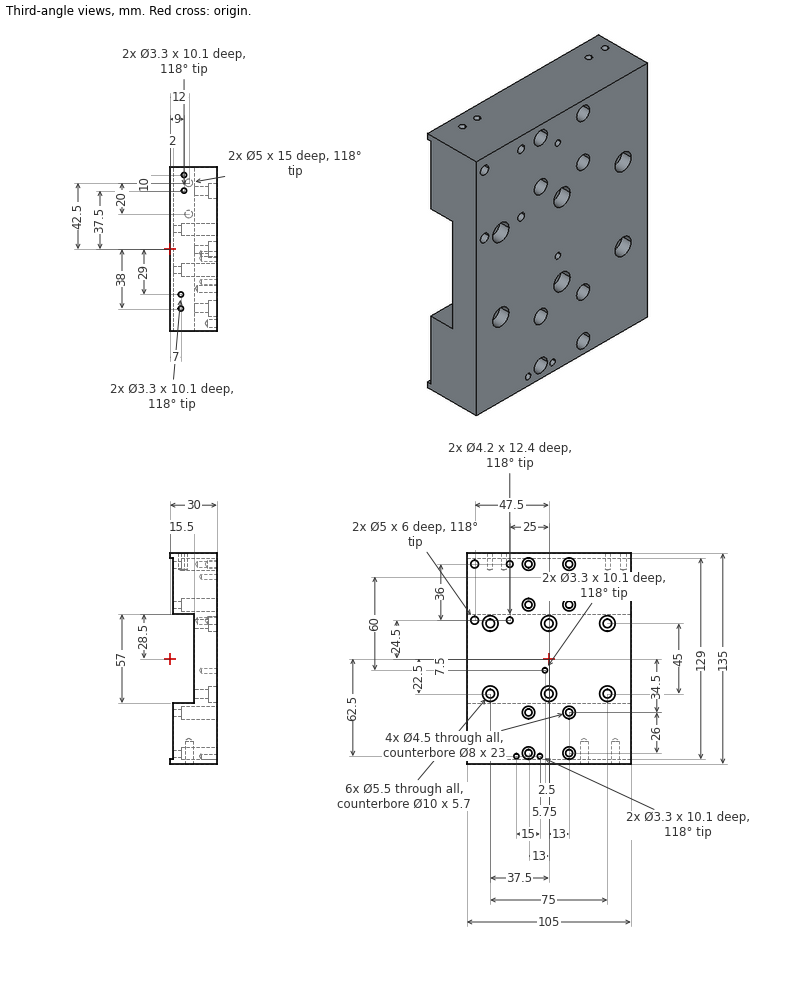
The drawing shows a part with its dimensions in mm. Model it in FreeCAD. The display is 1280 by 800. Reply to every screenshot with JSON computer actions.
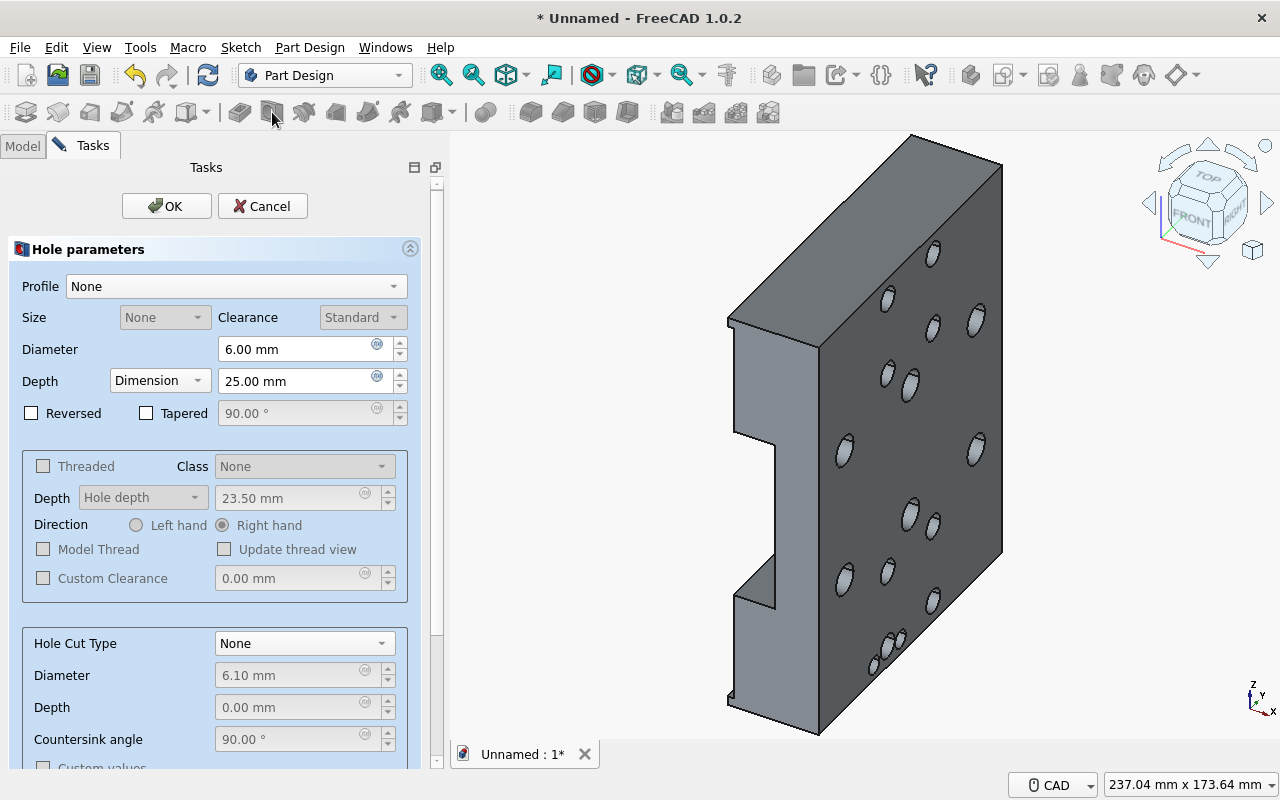
{"action": "triple_click", "coordinate": [305, 349]}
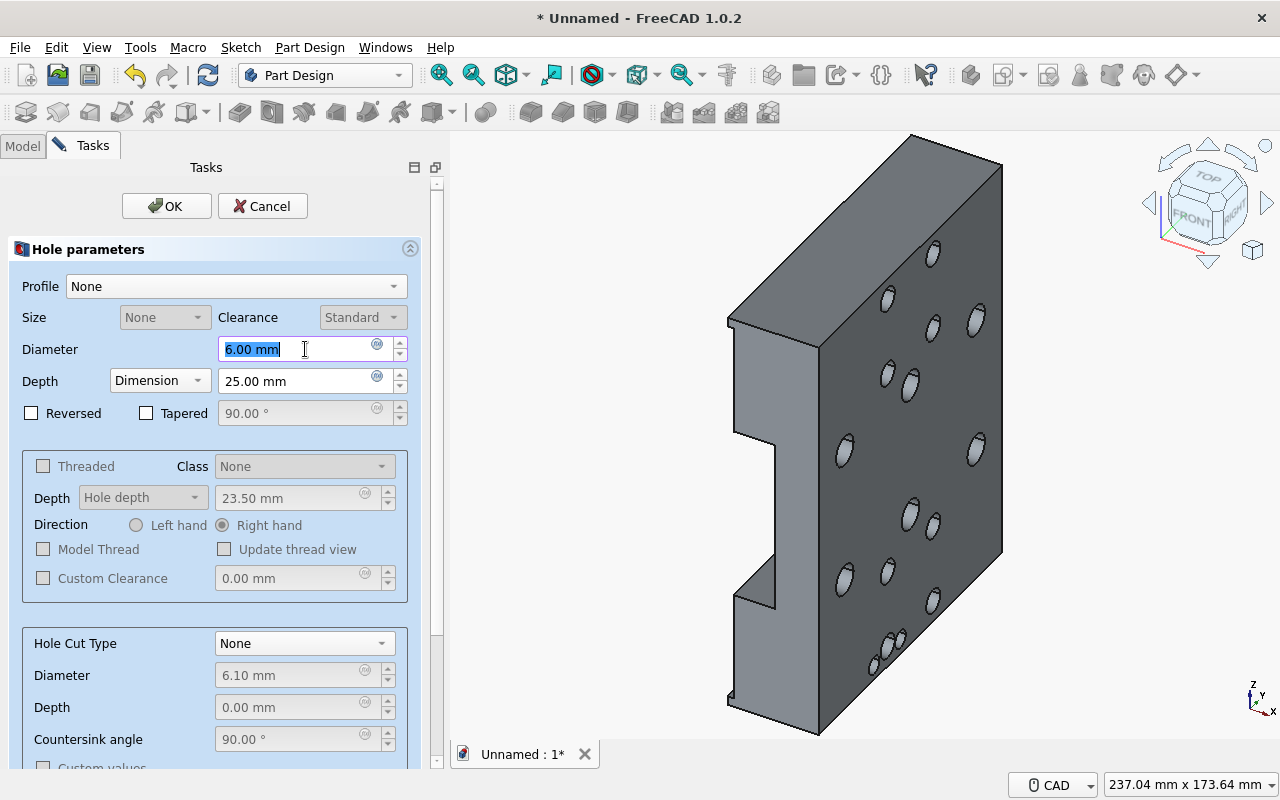
{"action": "type", "text": "3.3"}
{"action": "key", "text": "Tab"}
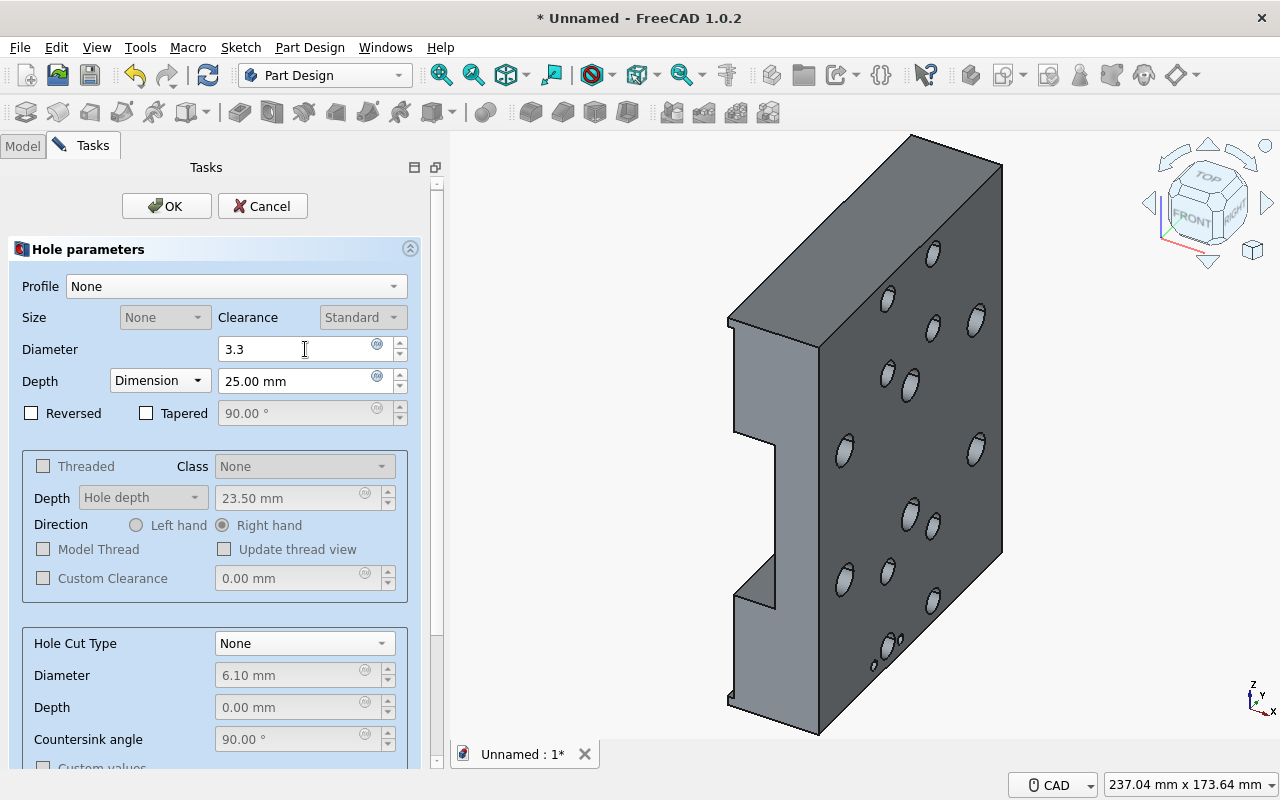
{"action": "triple_click", "coordinate": [305, 381]}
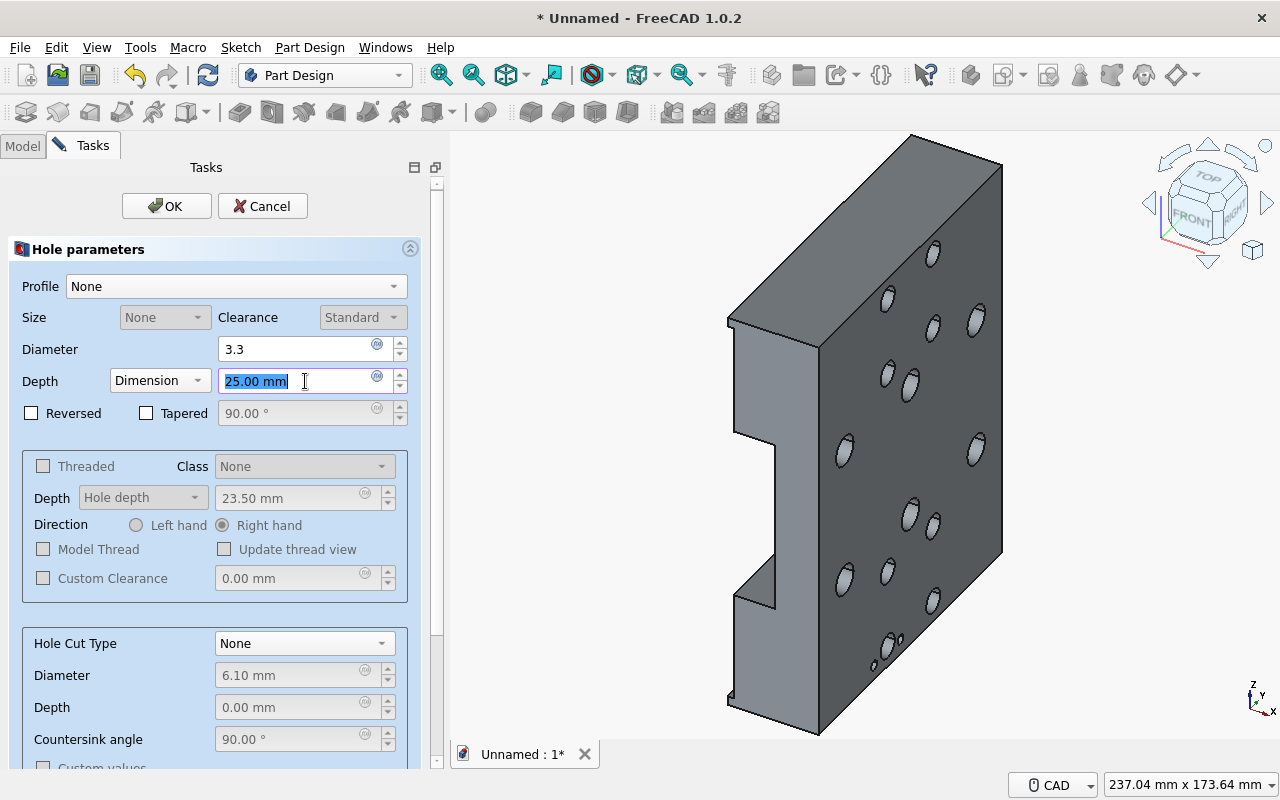
{"action": "type", "text": "10.1"}
{"action": "key", "text": "Tab"}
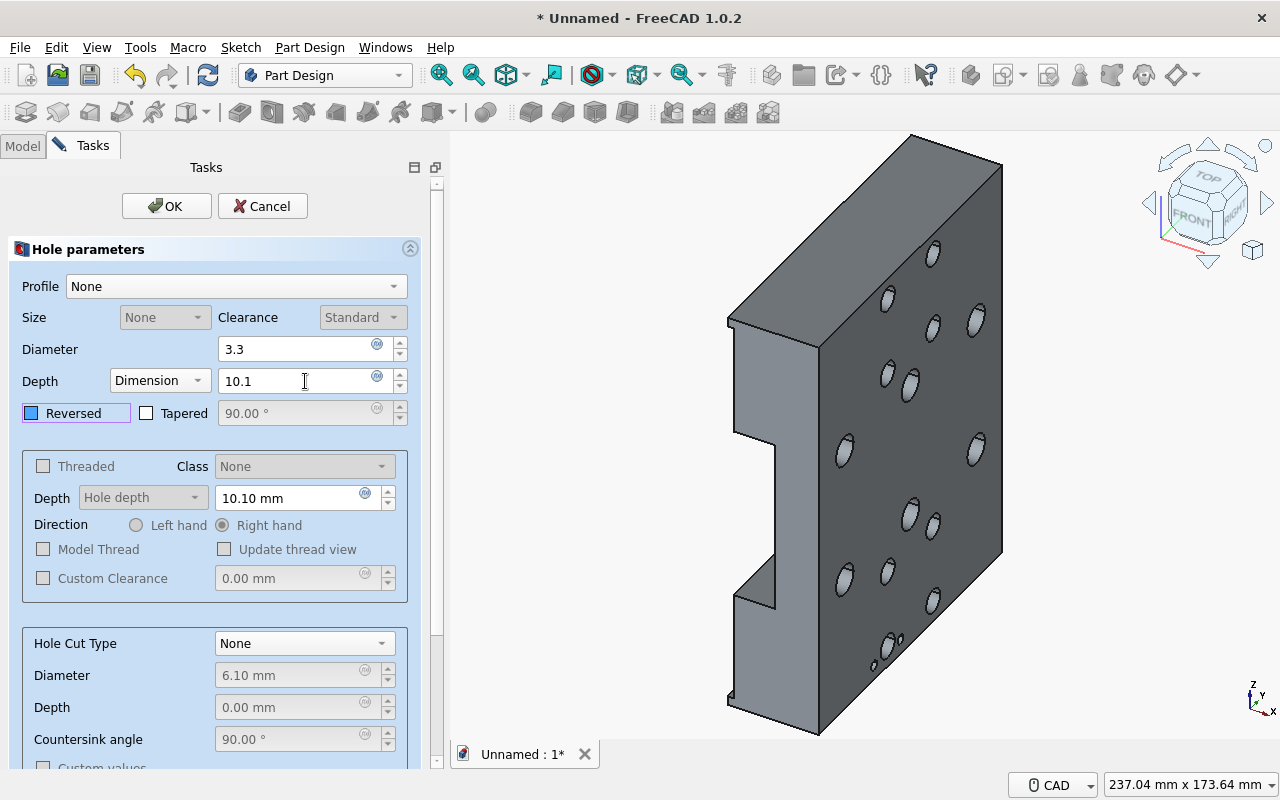
{"action": "left_click", "coordinate": [167, 206]}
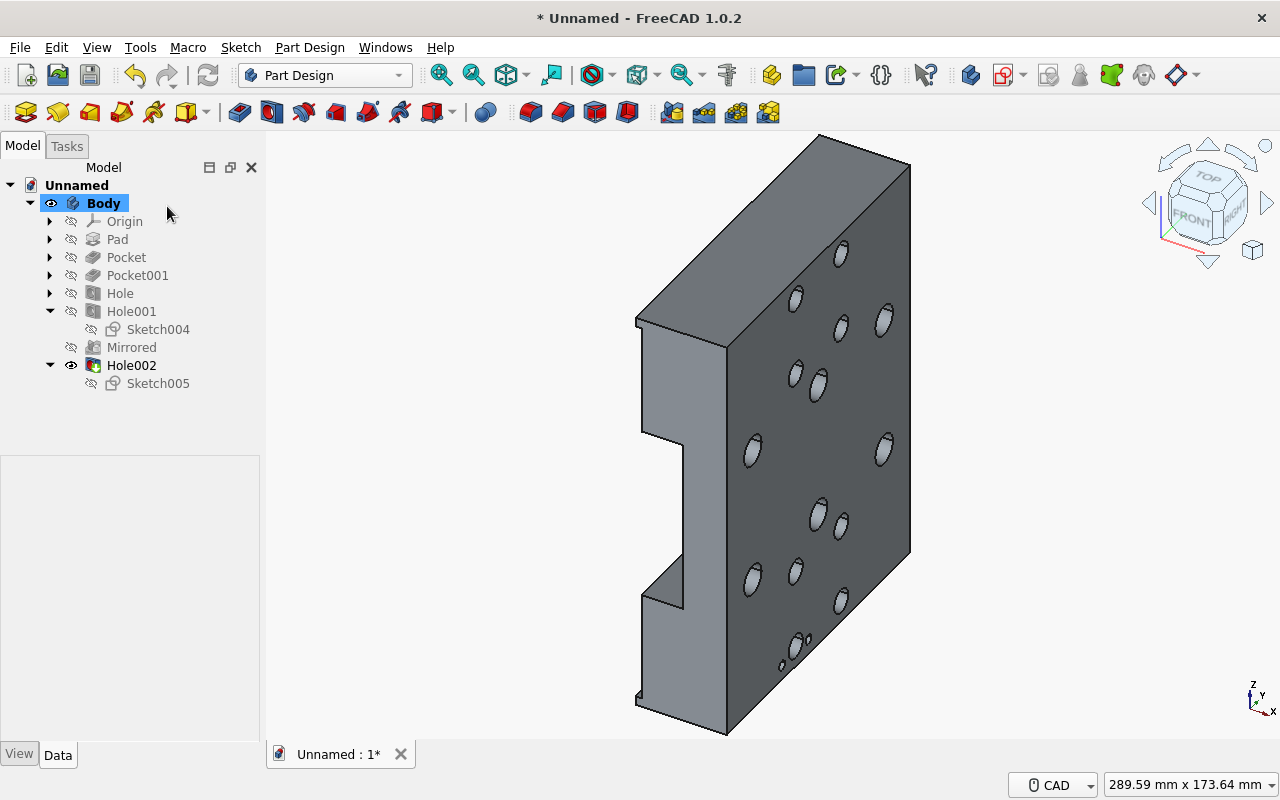
{"action": "key", "text": "5"}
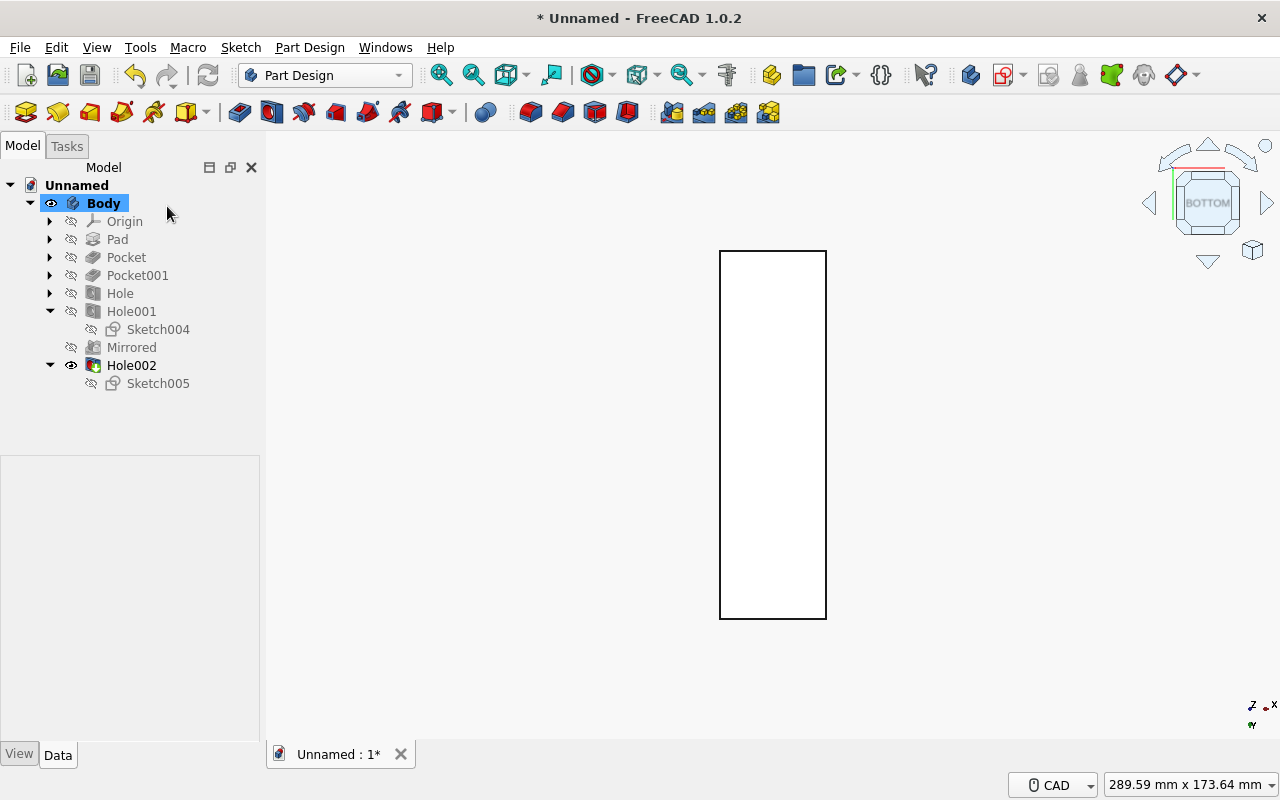
{"action": "left_click", "coordinate": [773, 539]}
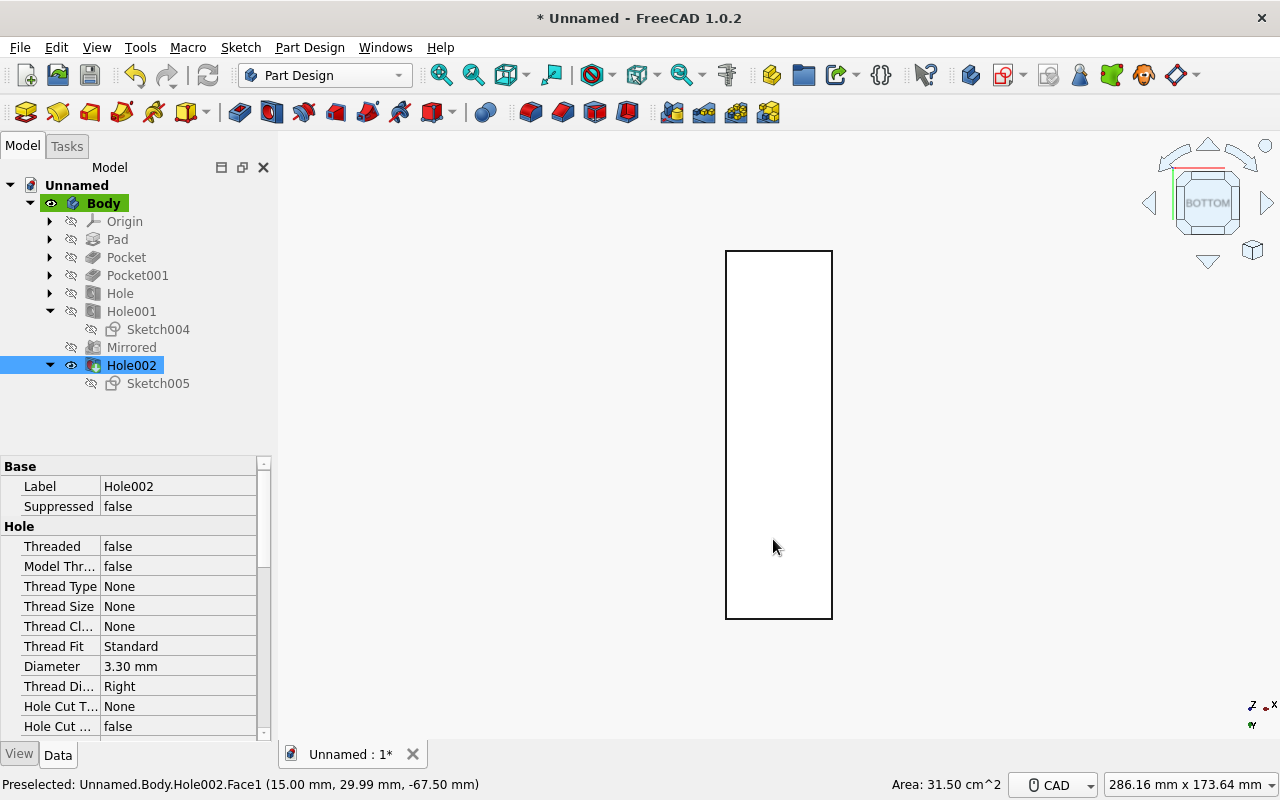
{"action": "left_click", "coordinate": [1004, 76]}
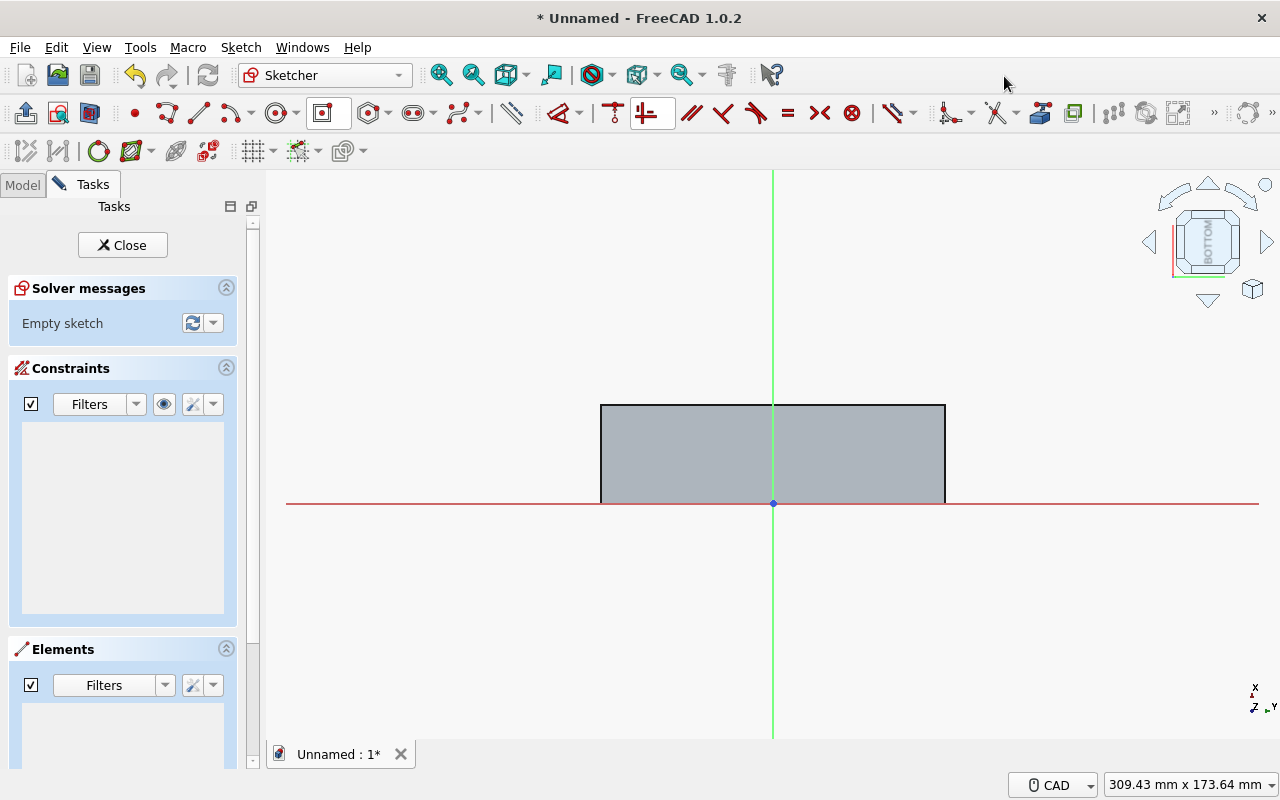
{"action": "scroll", "coordinate": [893, 488], "scroll_direction": "up", "scroll_amount": 7}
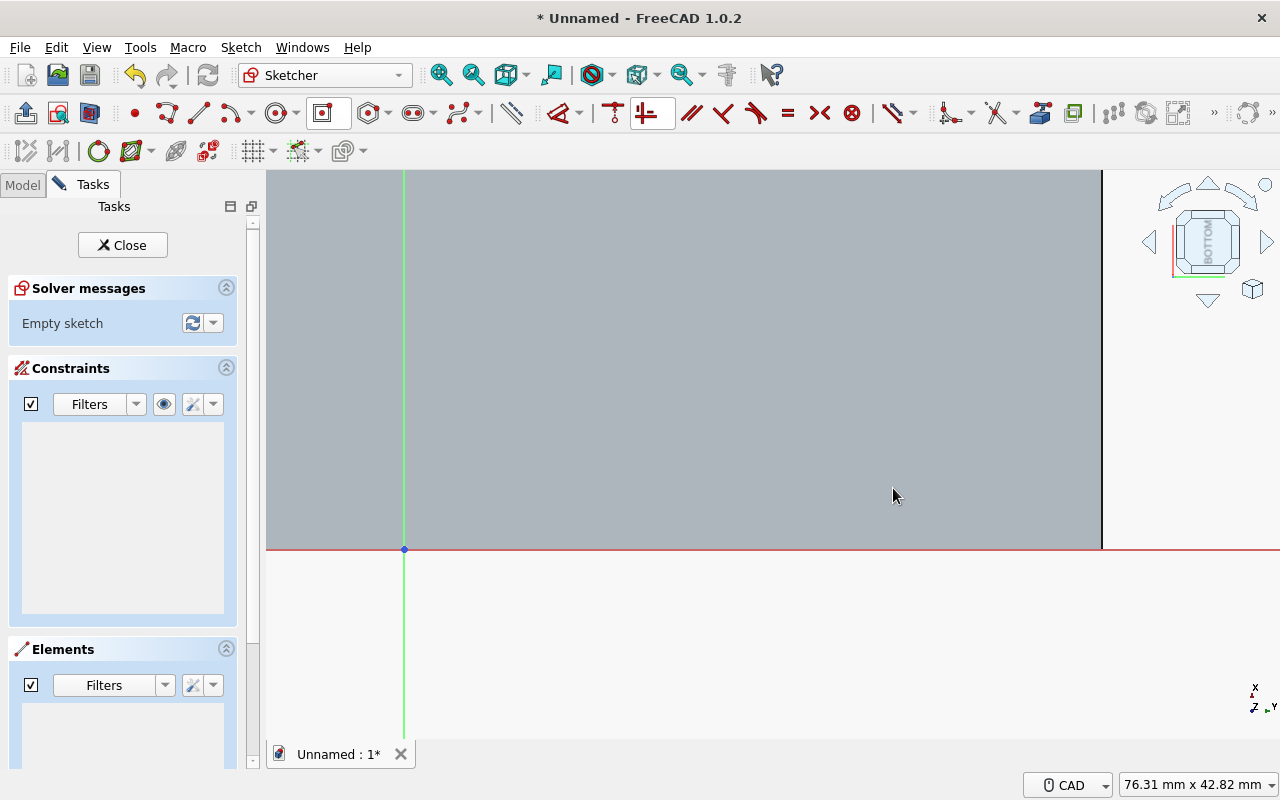
{"action": "left_click", "coordinate": [276, 114]}